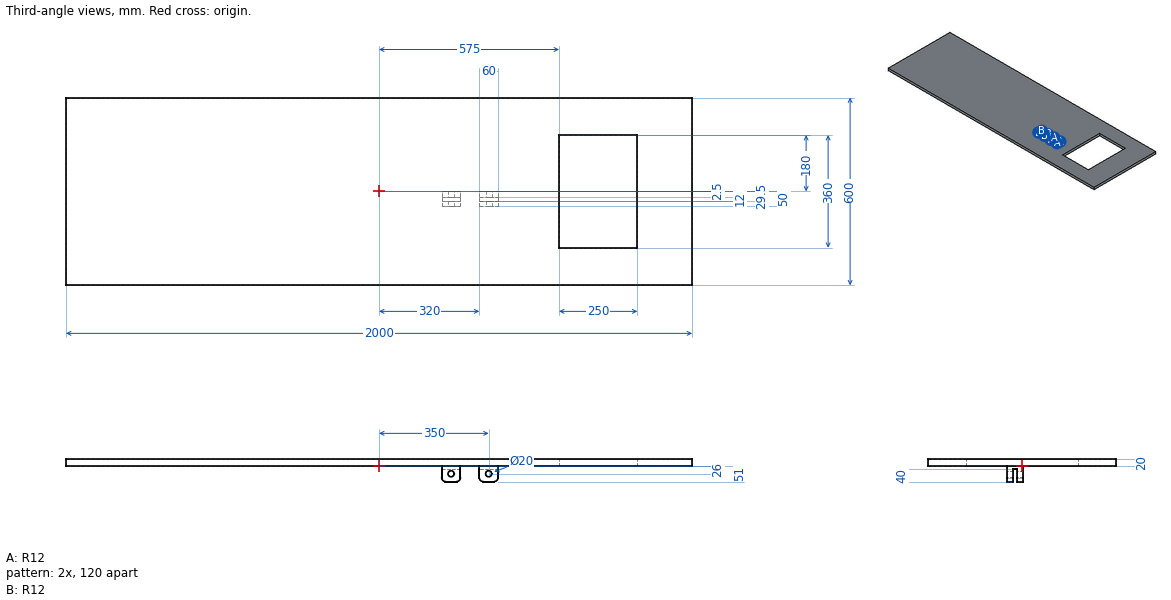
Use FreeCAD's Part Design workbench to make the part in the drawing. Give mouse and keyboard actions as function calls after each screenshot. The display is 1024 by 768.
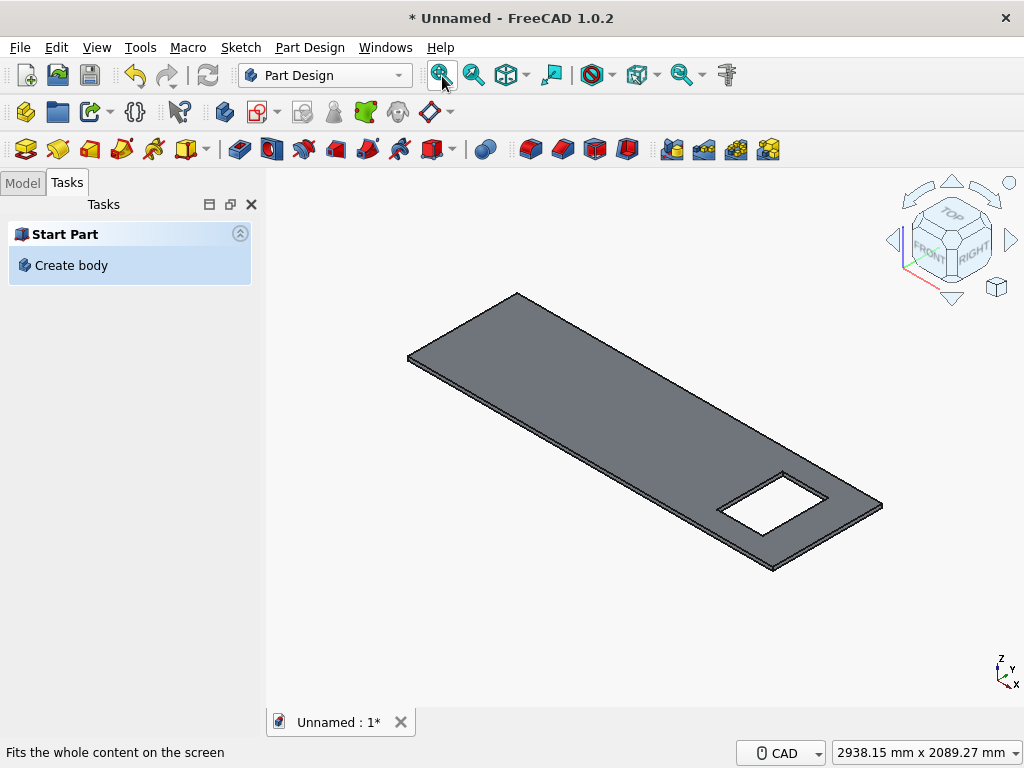
scroll(700, 480, up, 4)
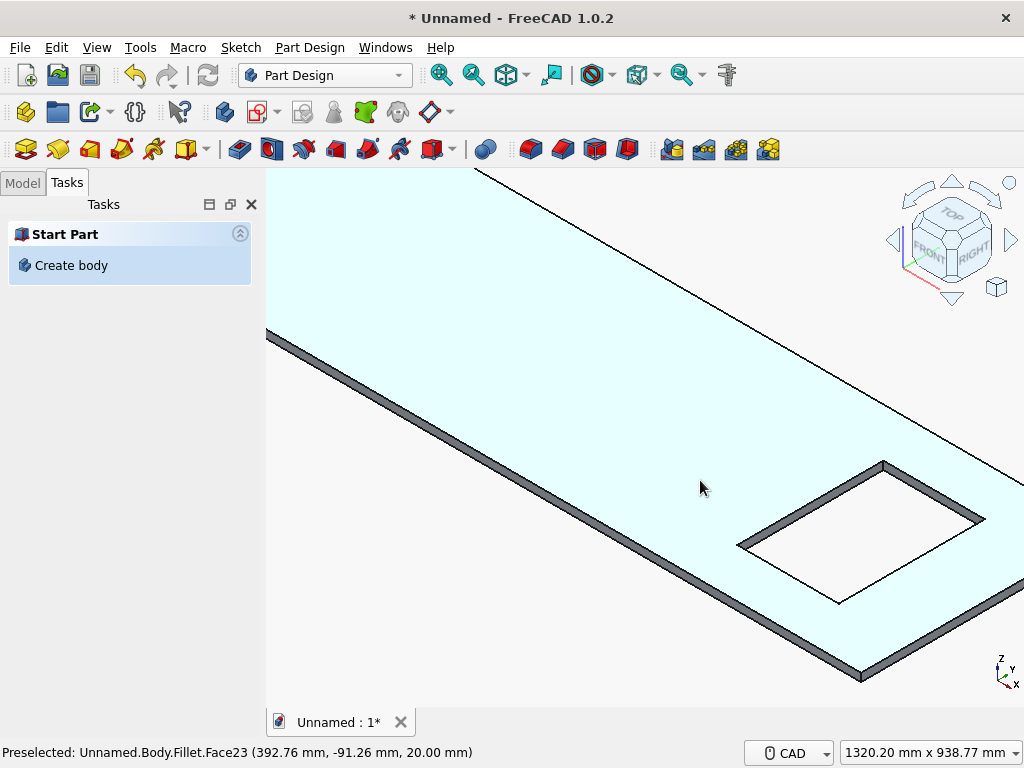
click(442, 76)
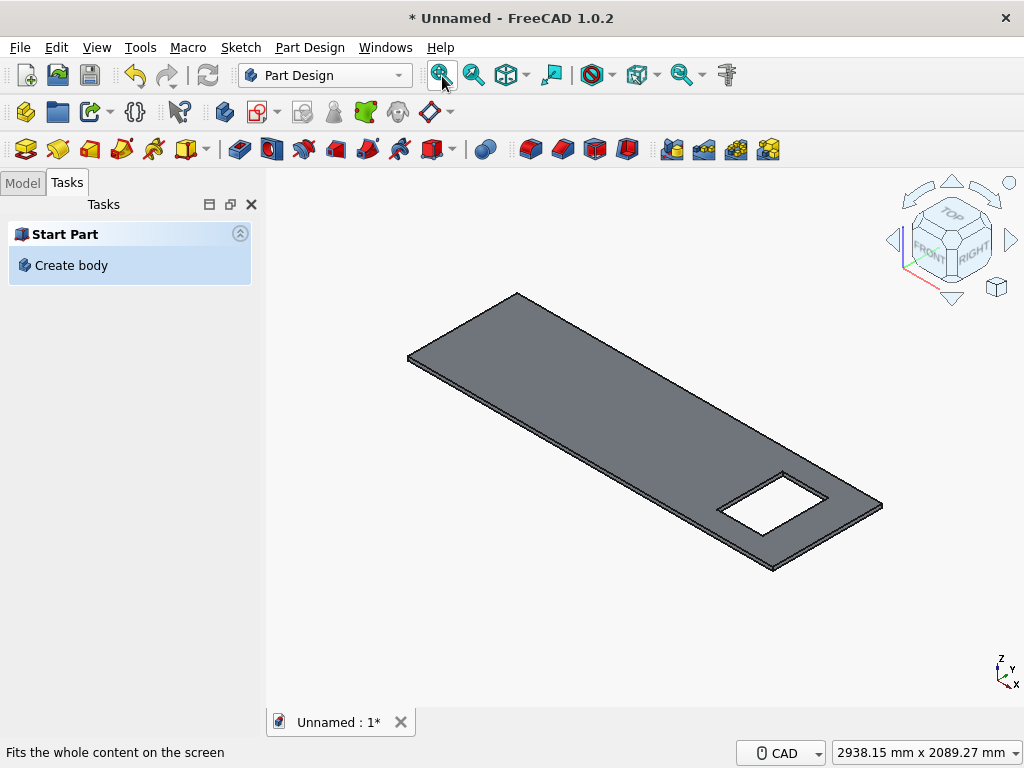
key(1)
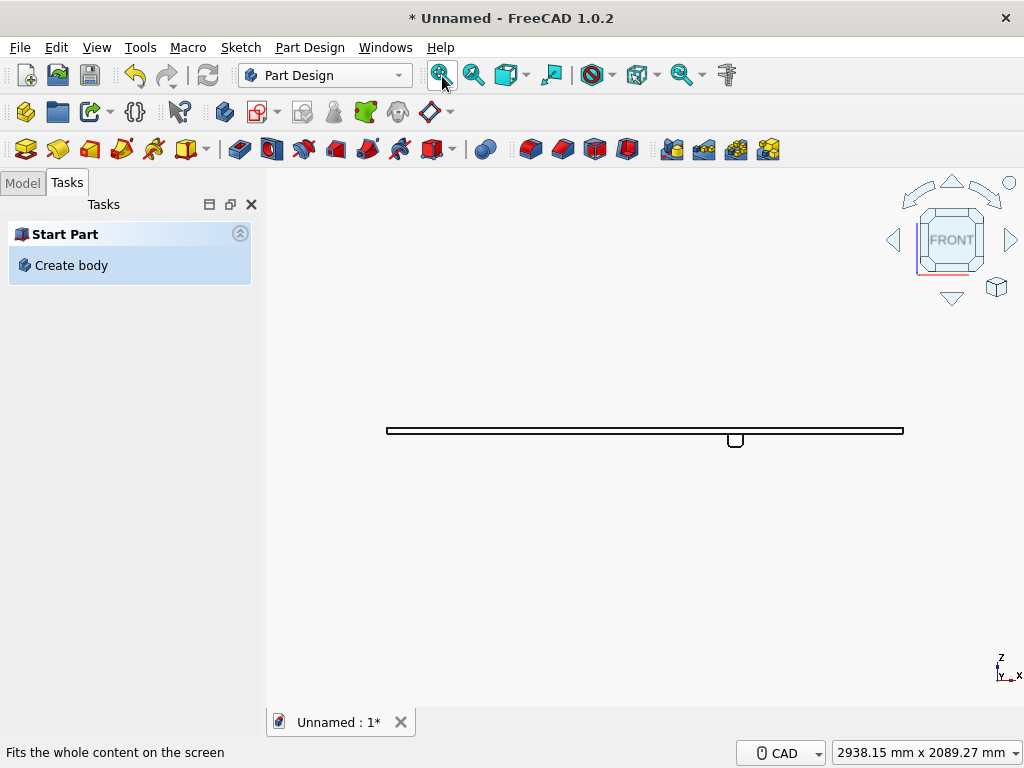
scroll(735, 439, up, 4)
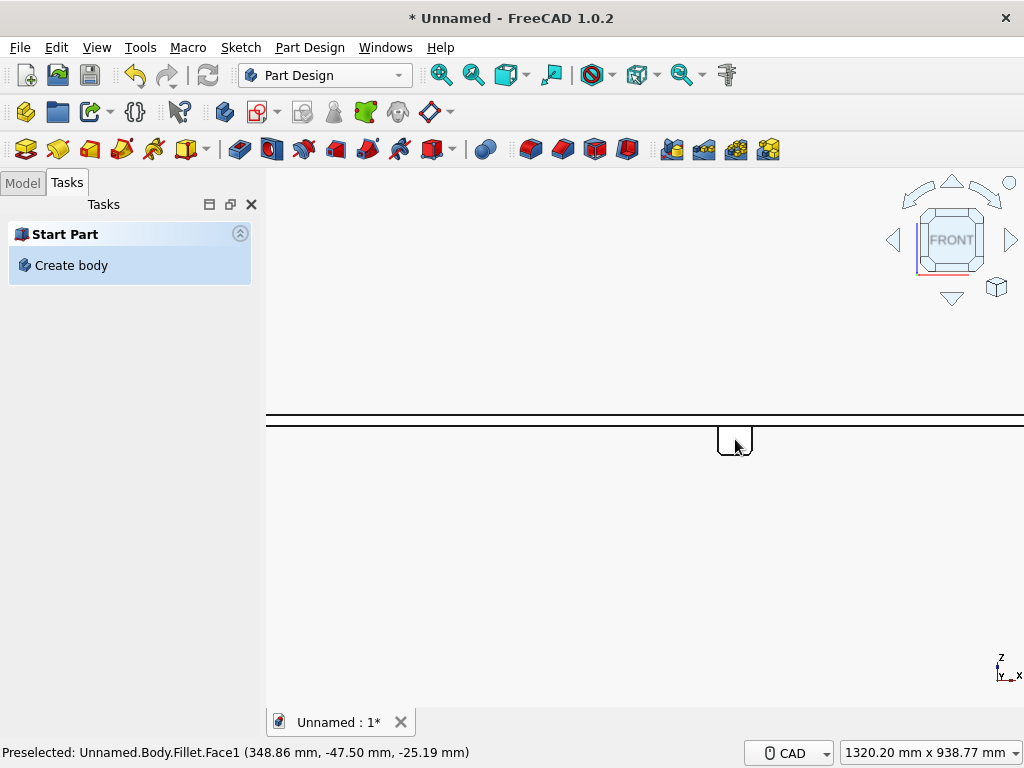
click(735, 440)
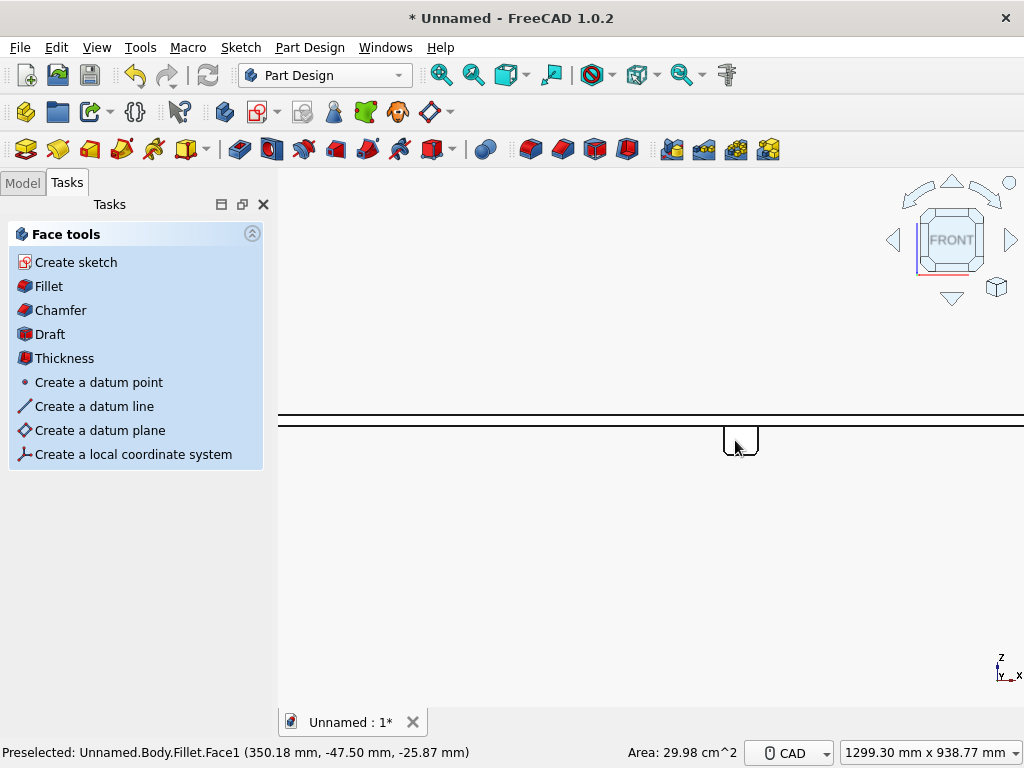
click(258, 112)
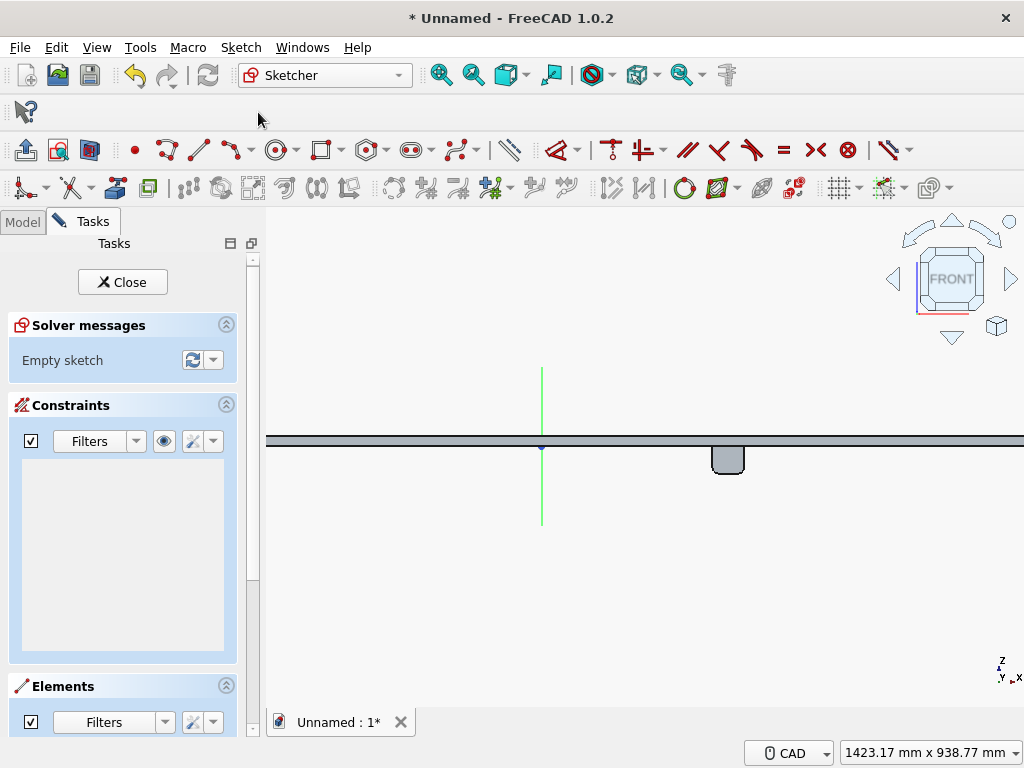
key(q)
key(s)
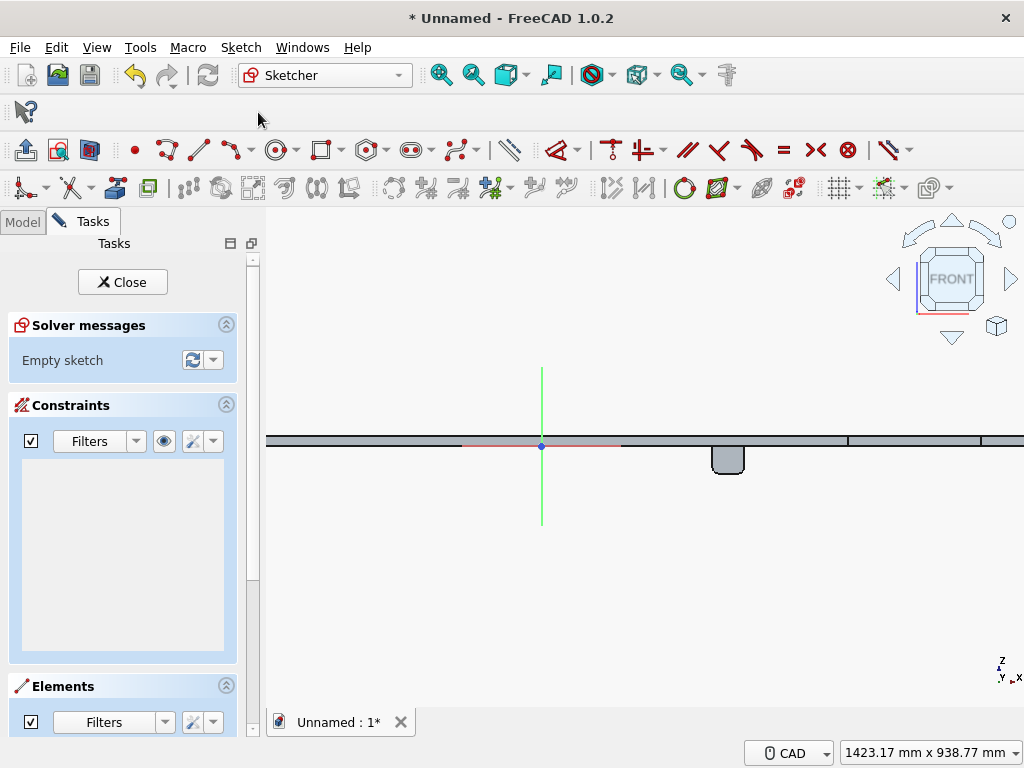
scroll(736, 460, up, 15)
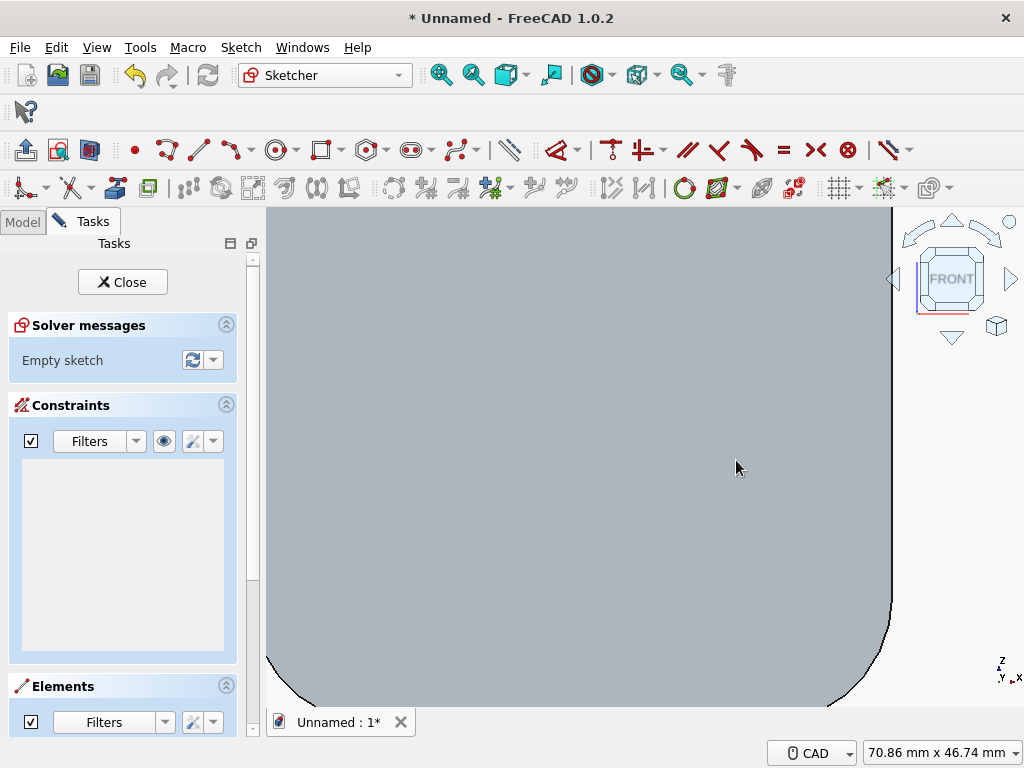
scroll(561, 456, up, 2)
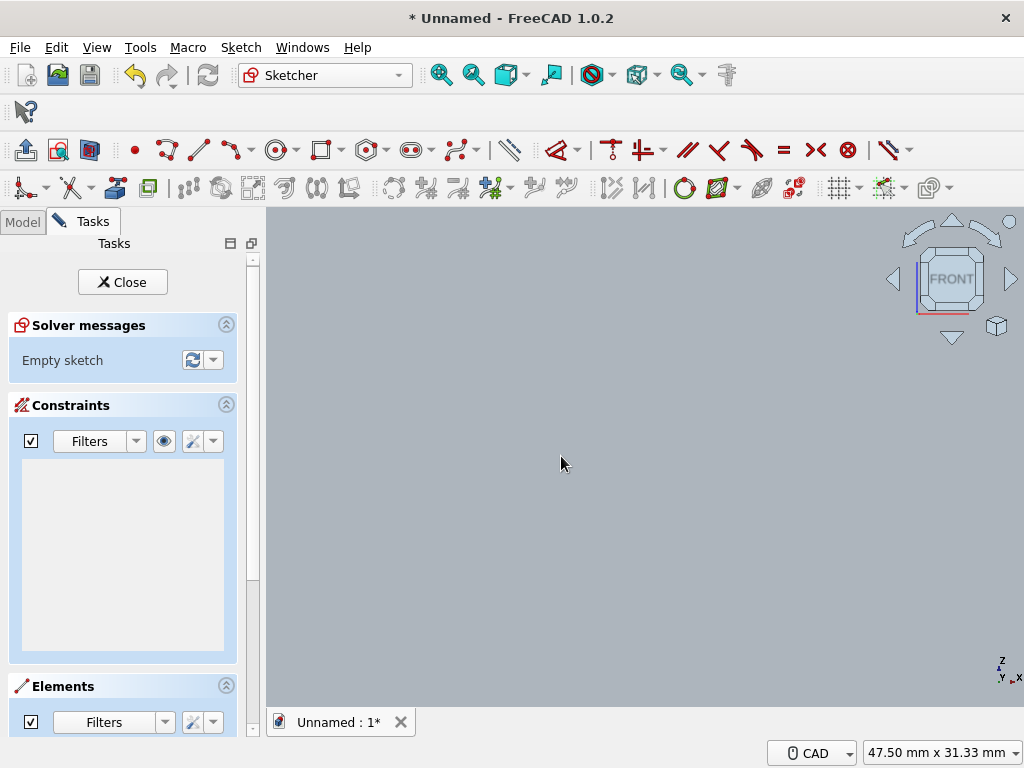
key(g)
key(c)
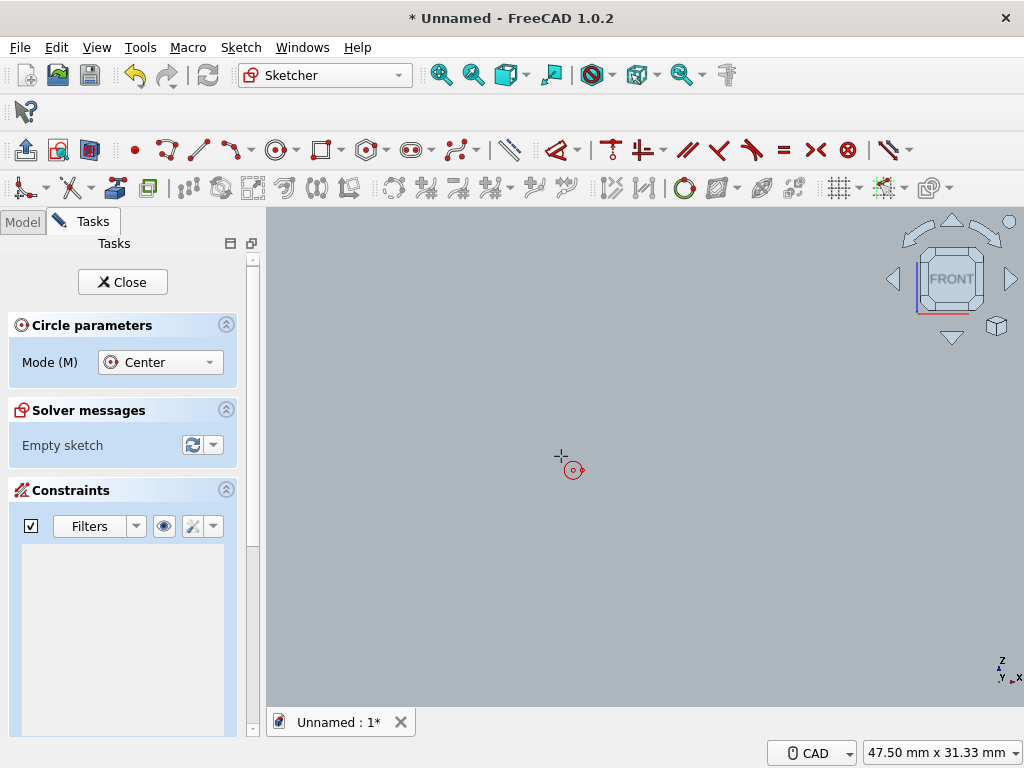
click(576, 457)
move(689, 344)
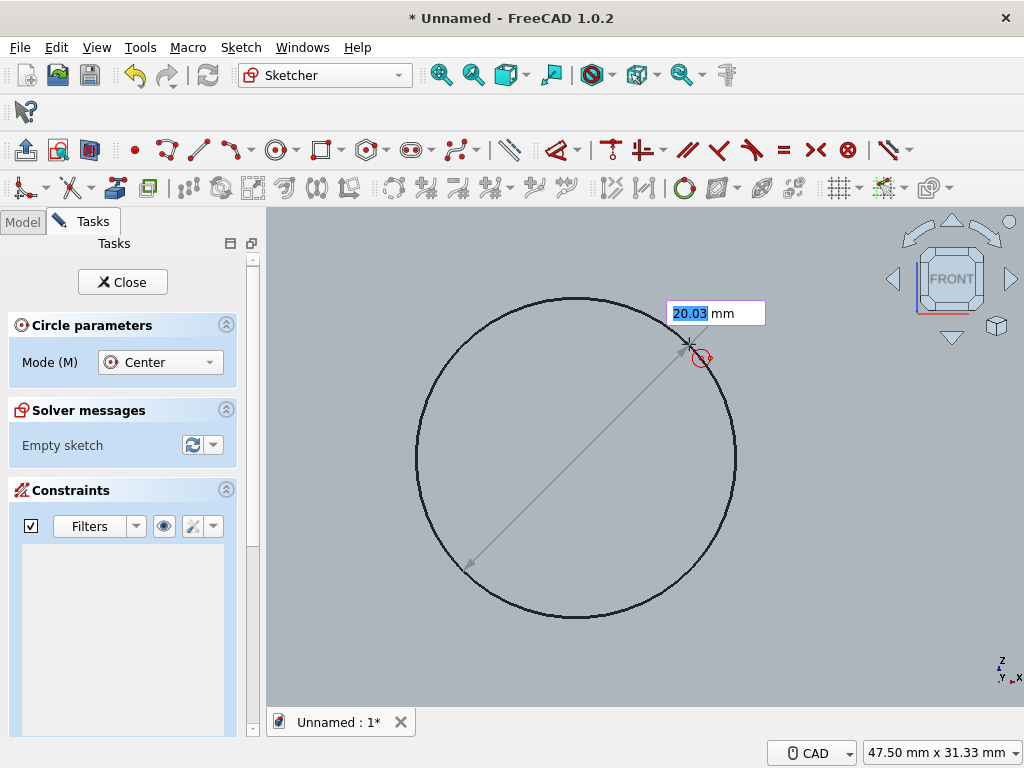
text(20)
key(Return)
key(Escape)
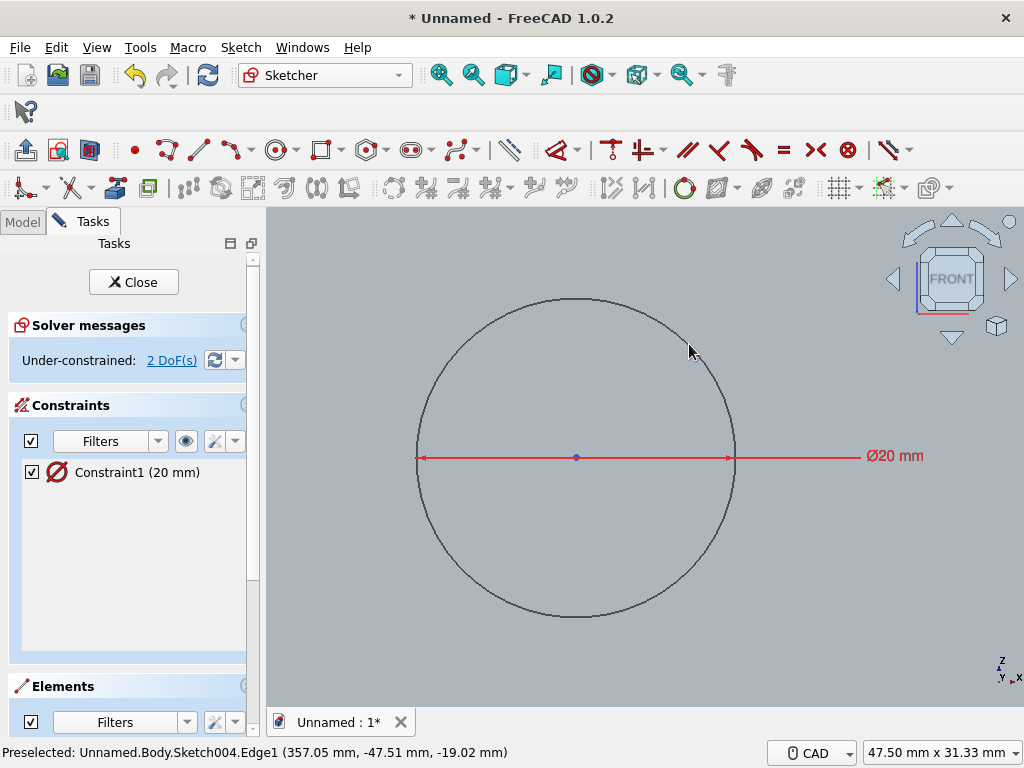
key(d)